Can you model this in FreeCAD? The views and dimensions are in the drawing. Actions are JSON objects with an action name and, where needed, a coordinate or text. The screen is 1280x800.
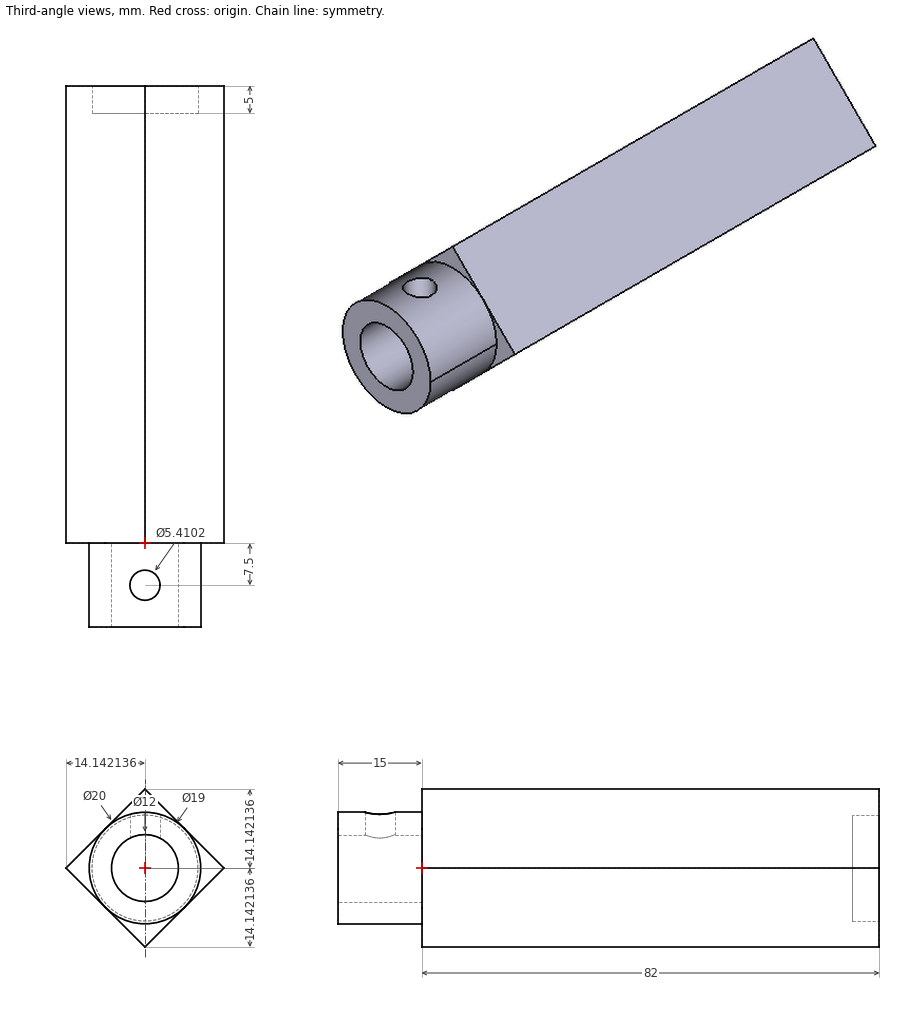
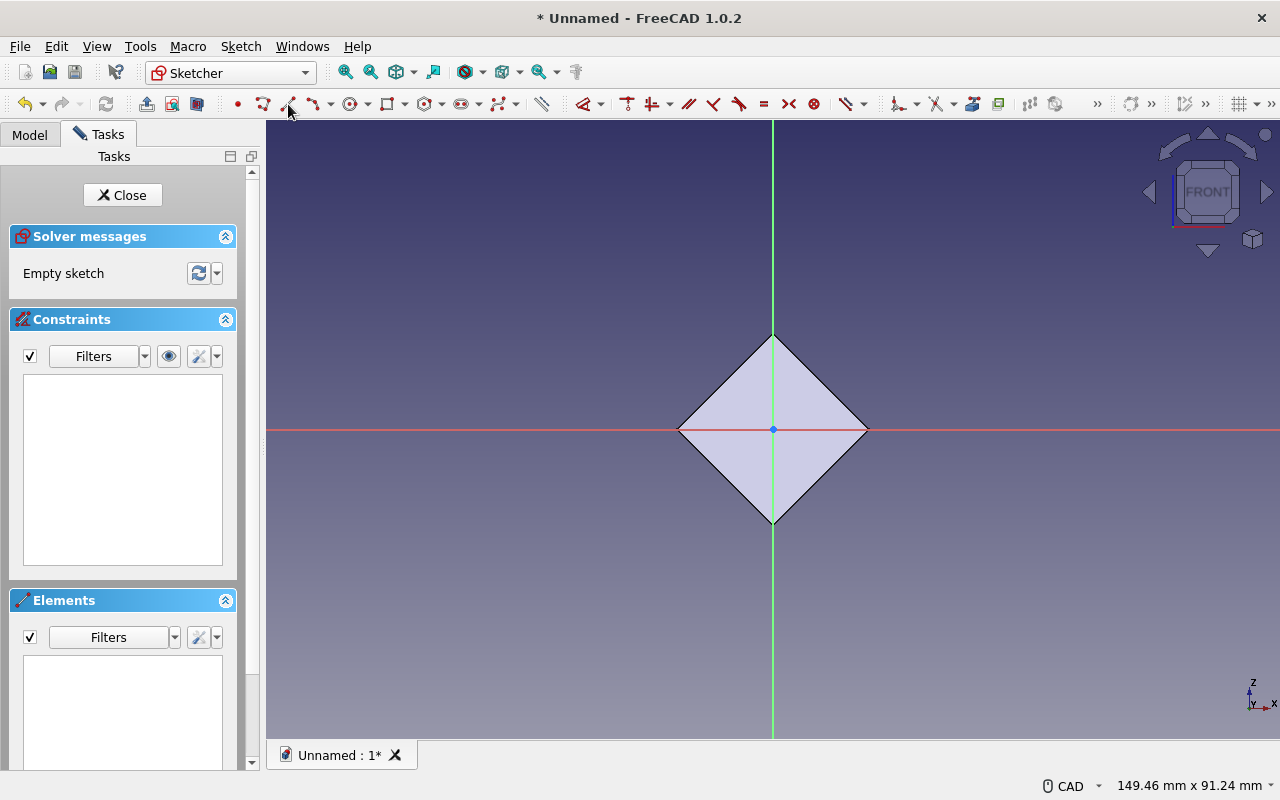
{"action": "scroll", "coordinate": [813, 430], "scroll_direction": "up", "scroll_amount": 5}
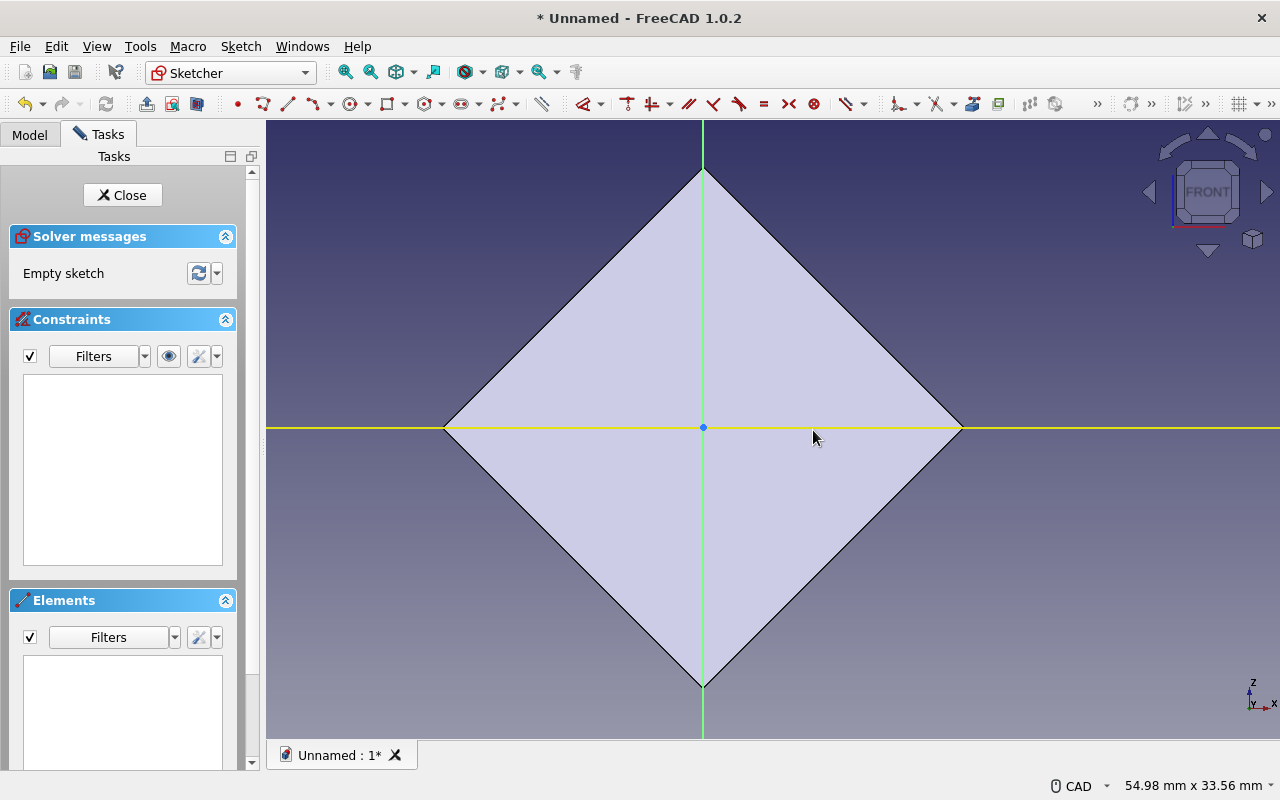
{"action": "key", "text": "g c"}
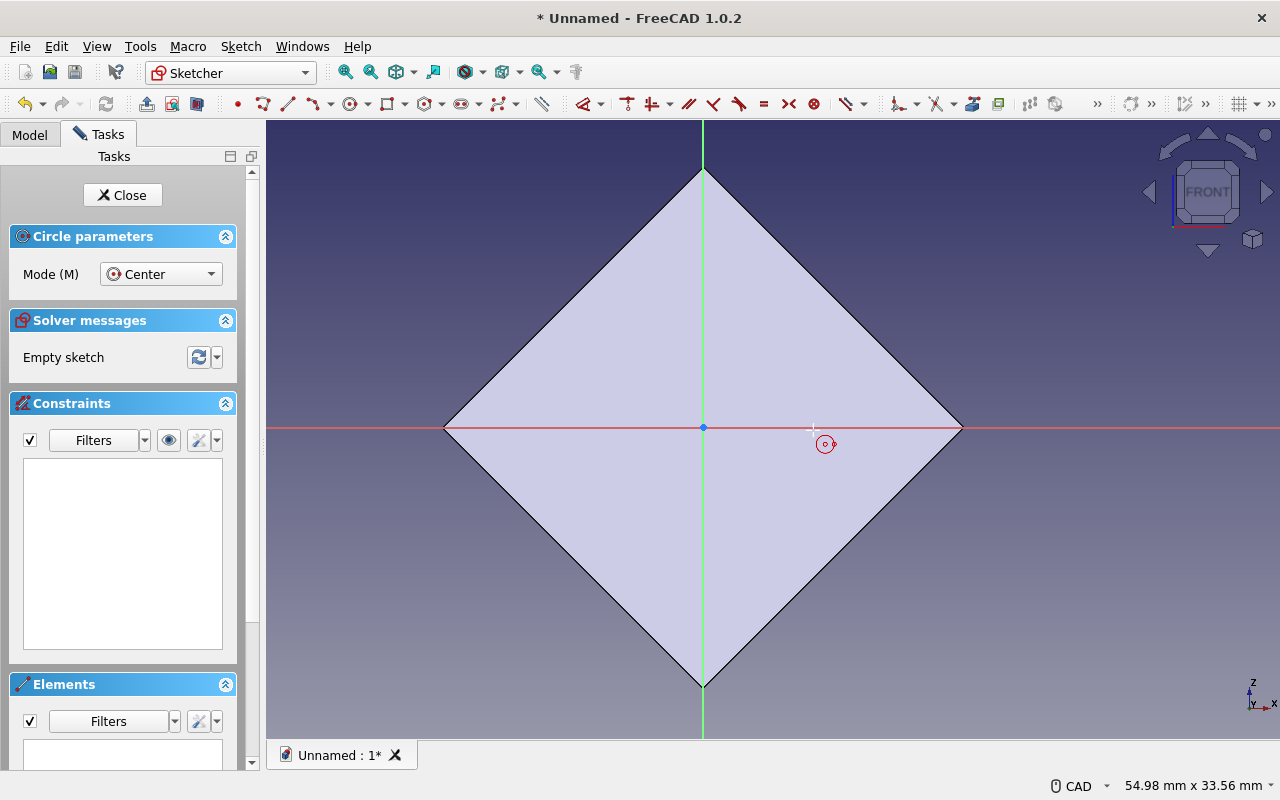
{"action": "left_click", "coordinate": [703, 428]}
{"action": "mouse_move", "coordinate": [834, 297]}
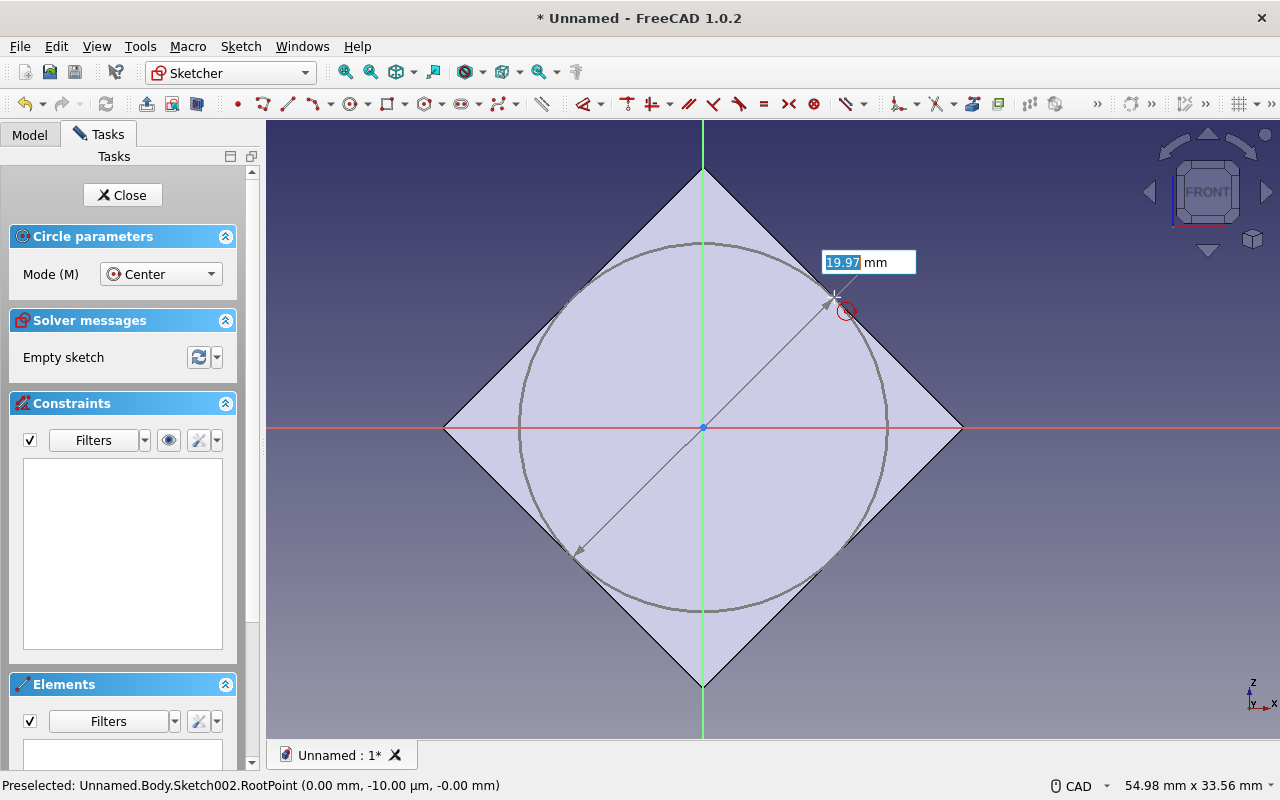
{"action": "type", "text": "20"}
{"action": "key", "text": "Return"}
{"action": "key", "text": "Escape"}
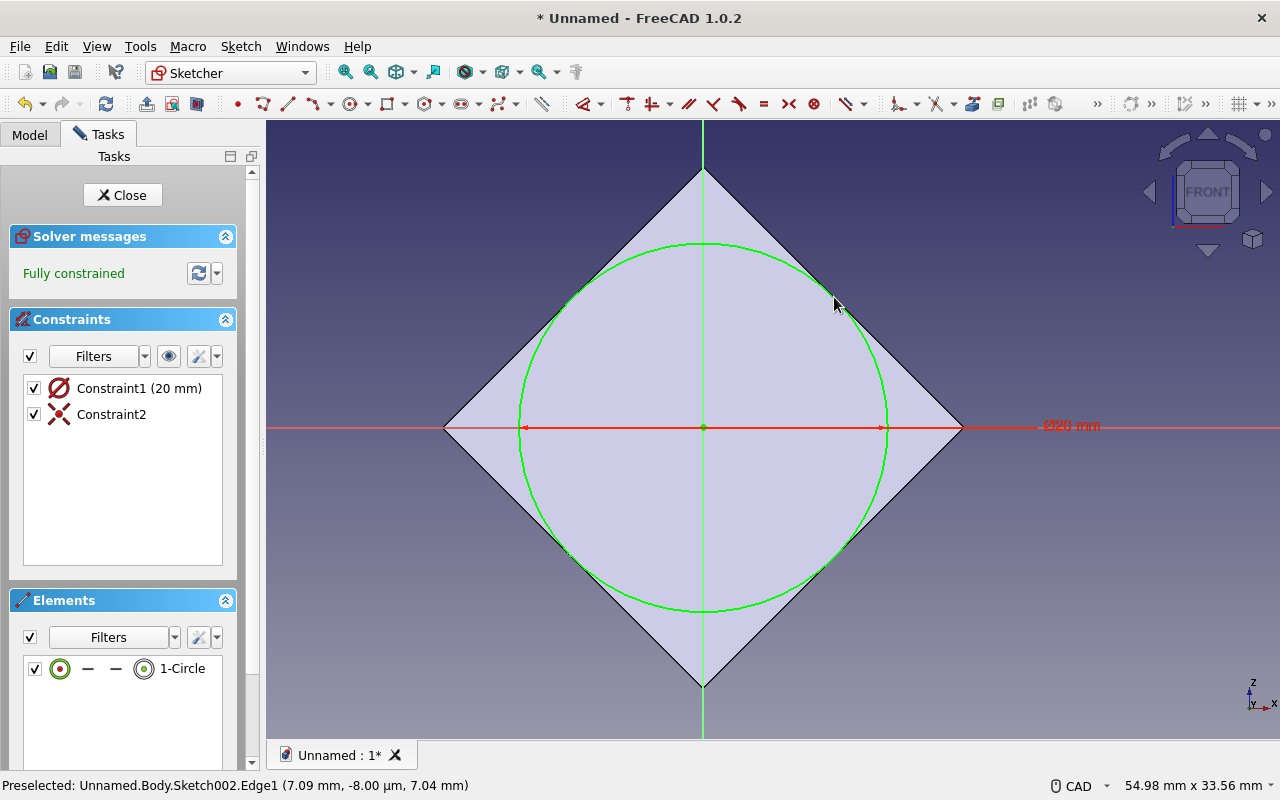
{"action": "left_click", "coordinate": [123, 195]}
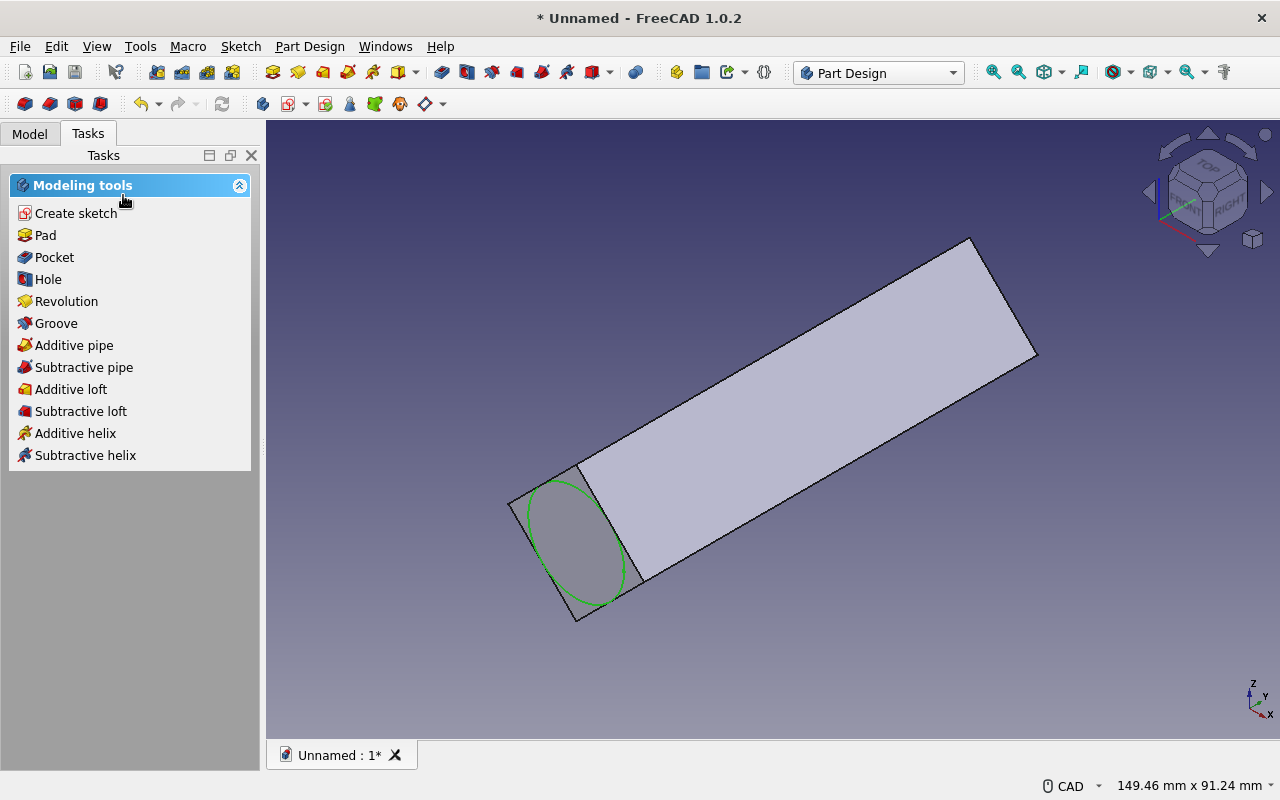
{"action": "left_click", "coordinate": [273, 72]}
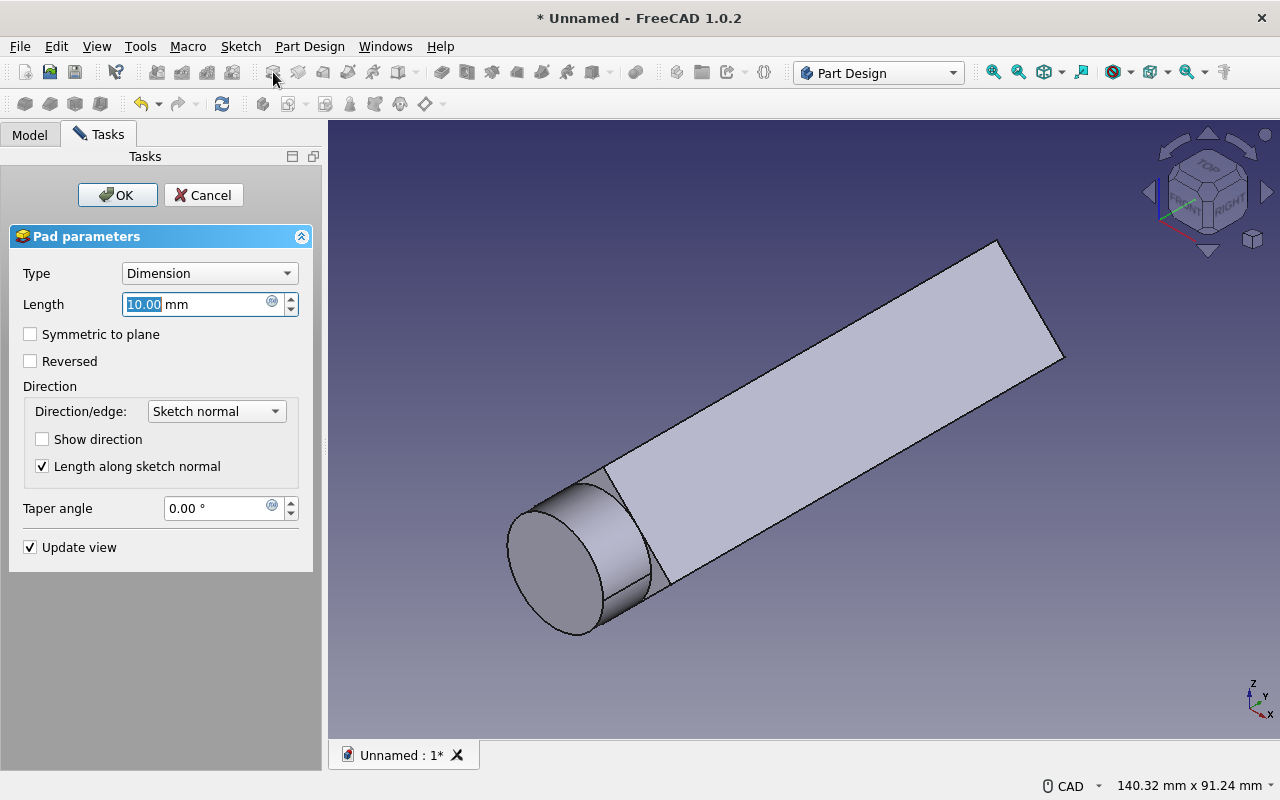
{"action": "type", "text": "15"}
{"action": "key", "text": "Tab"}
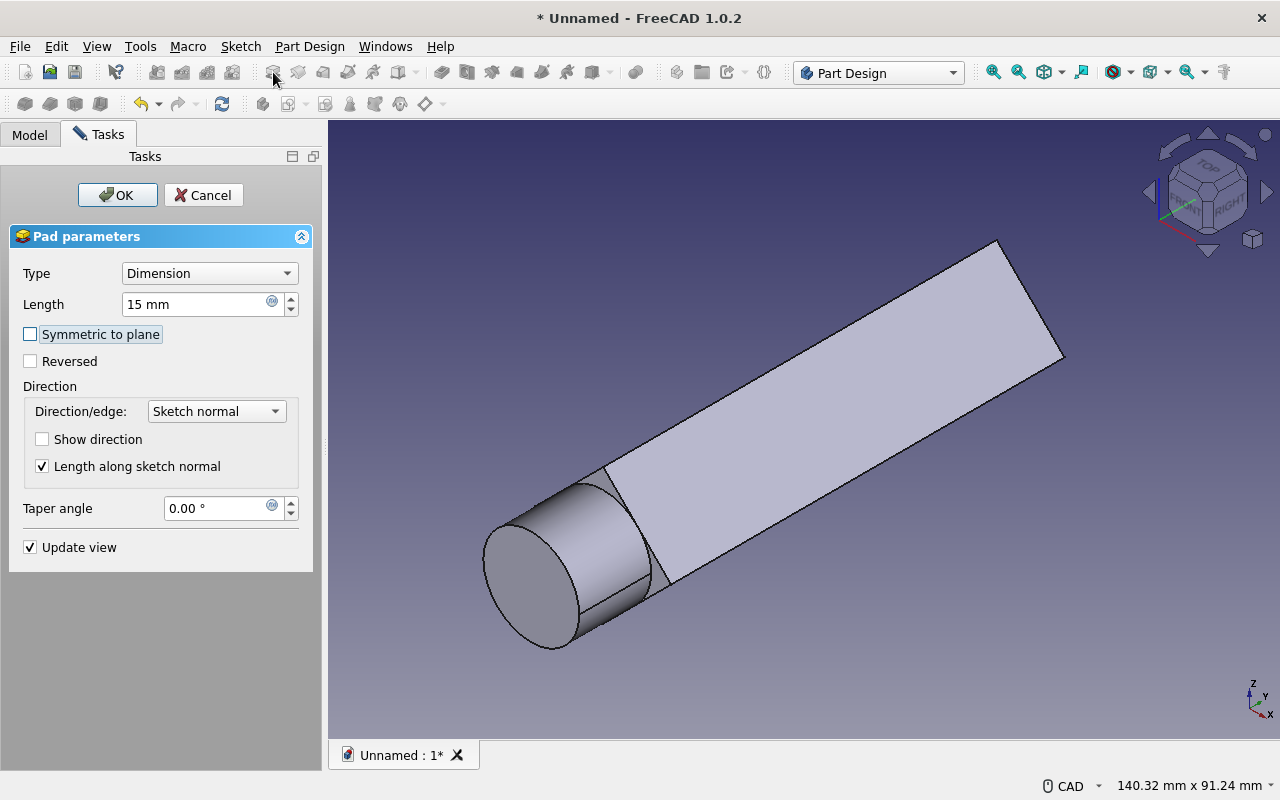
{"action": "left_click", "coordinate": [118, 195]}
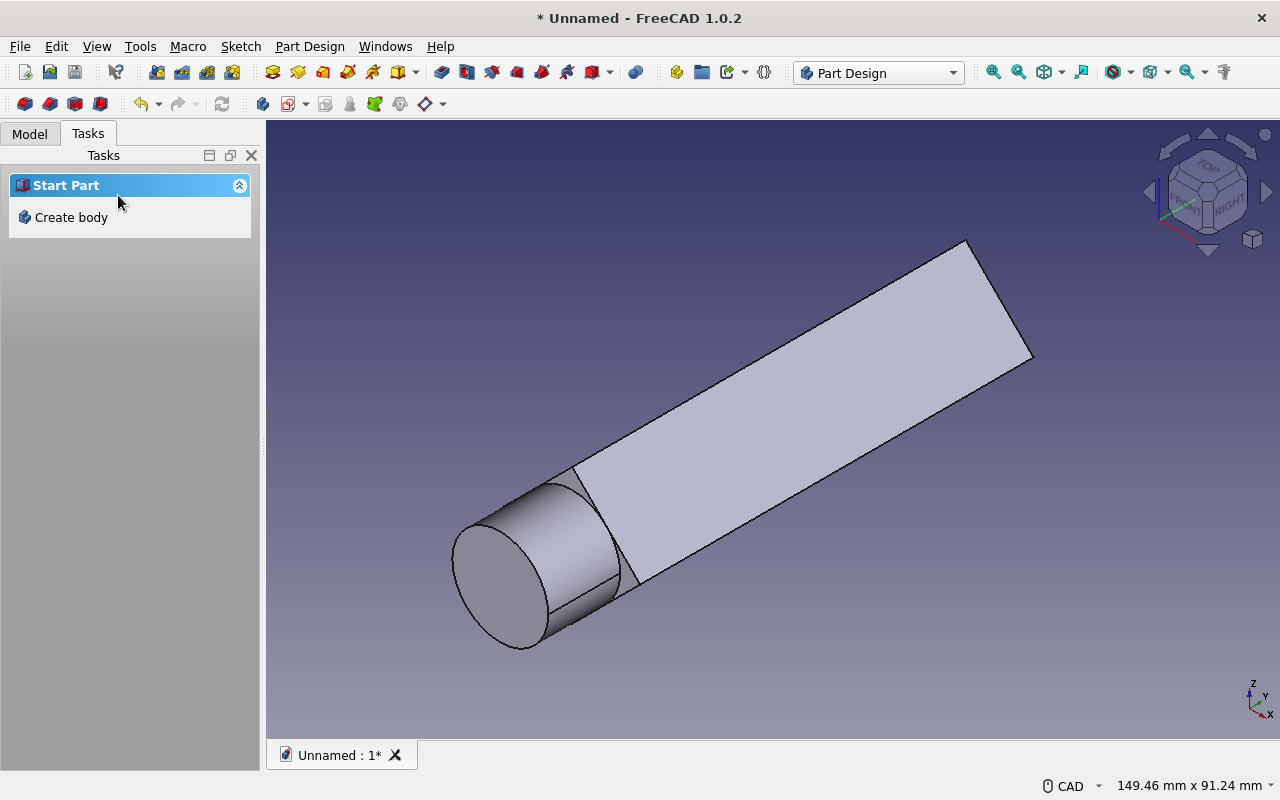
{"action": "left_click", "coordinate": [288, 104]}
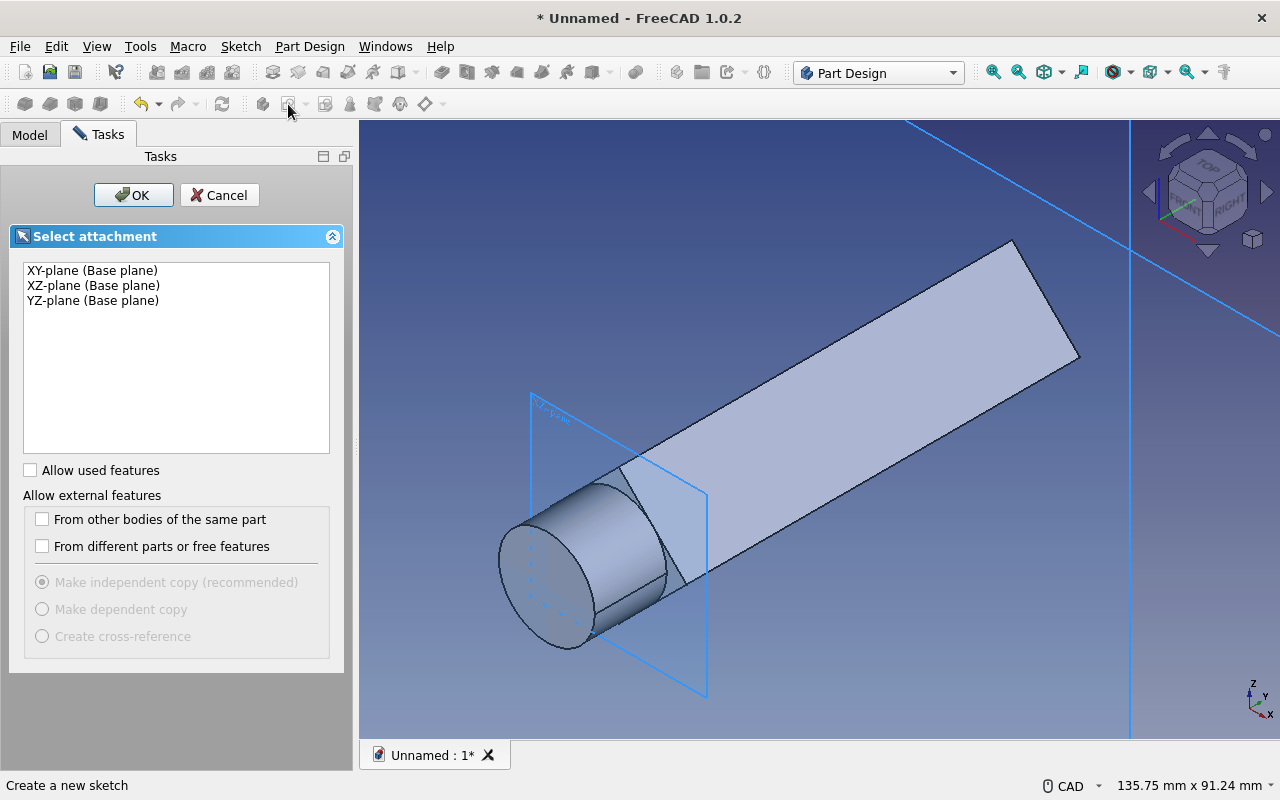
{"action": "left_click", "coordinate": [84, 286]}